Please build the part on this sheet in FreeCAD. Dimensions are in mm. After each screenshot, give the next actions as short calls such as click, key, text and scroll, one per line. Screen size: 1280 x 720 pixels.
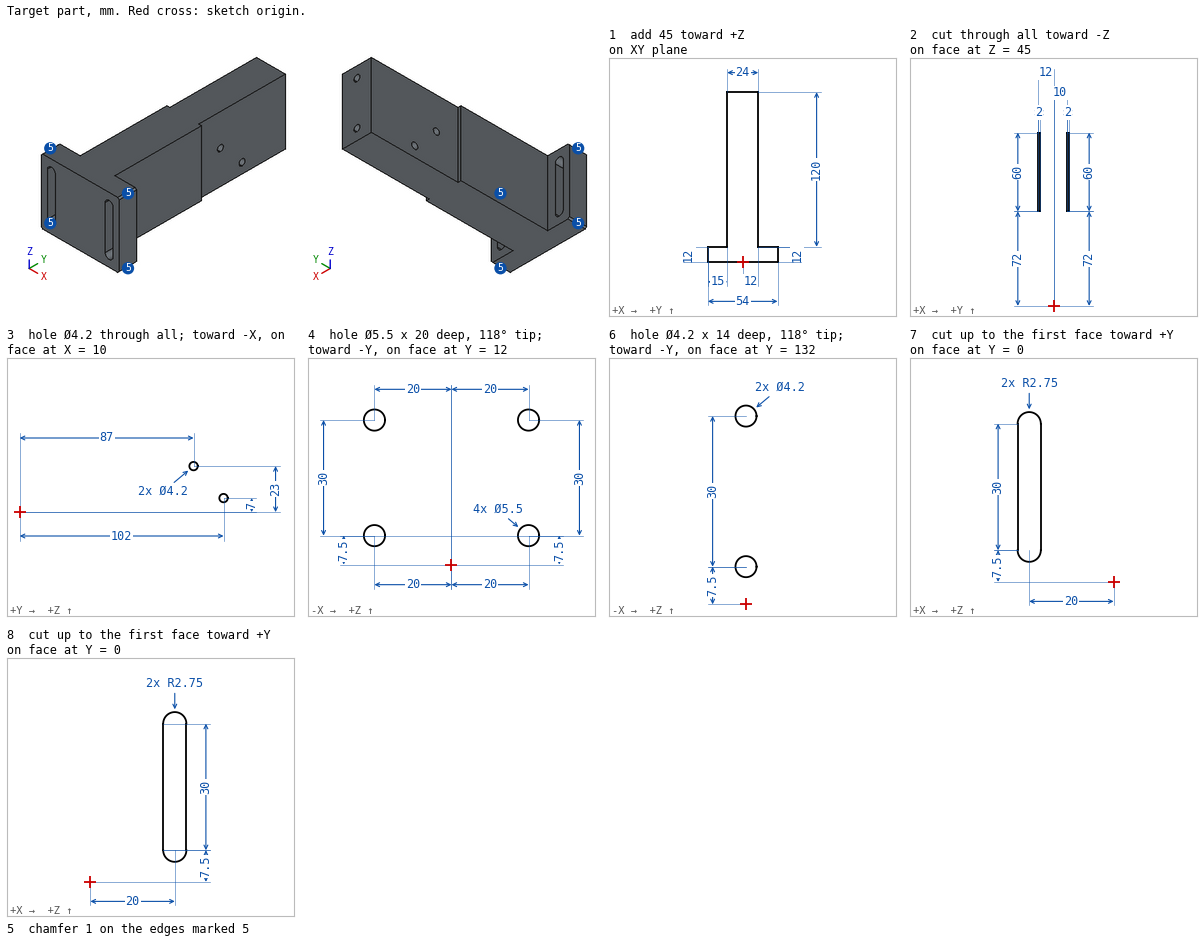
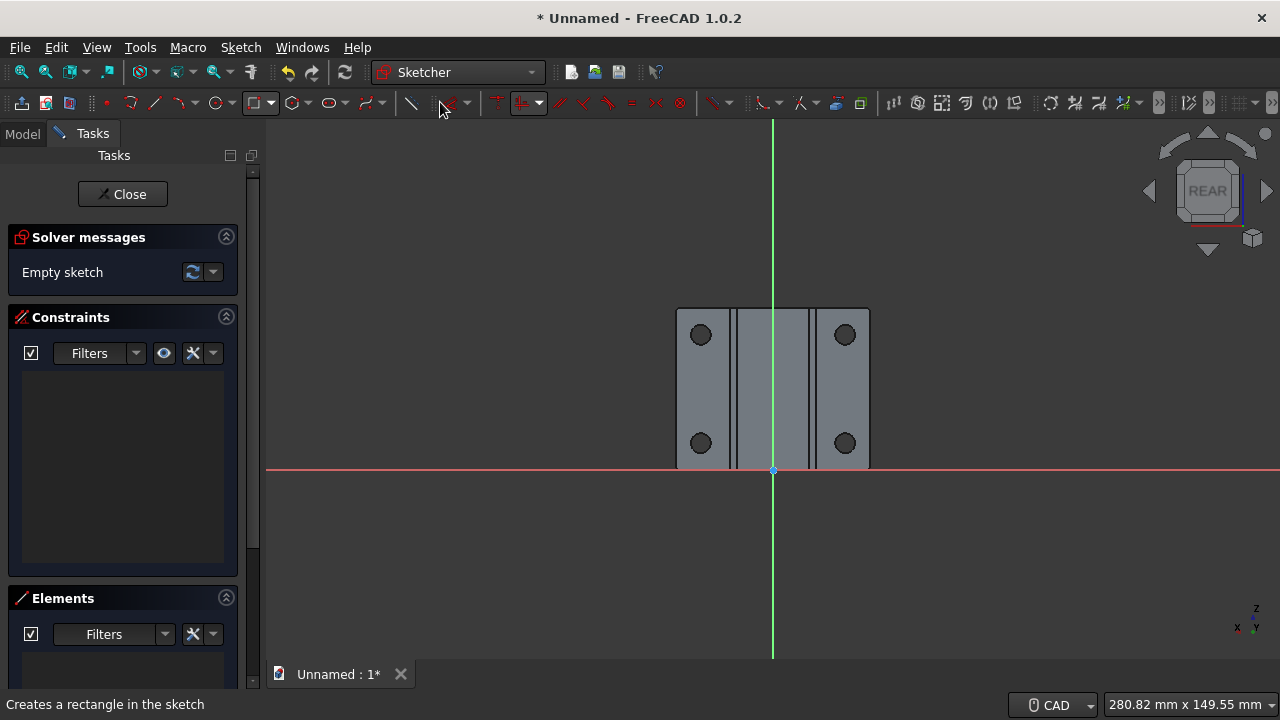
scroll(829, 407, up, 4)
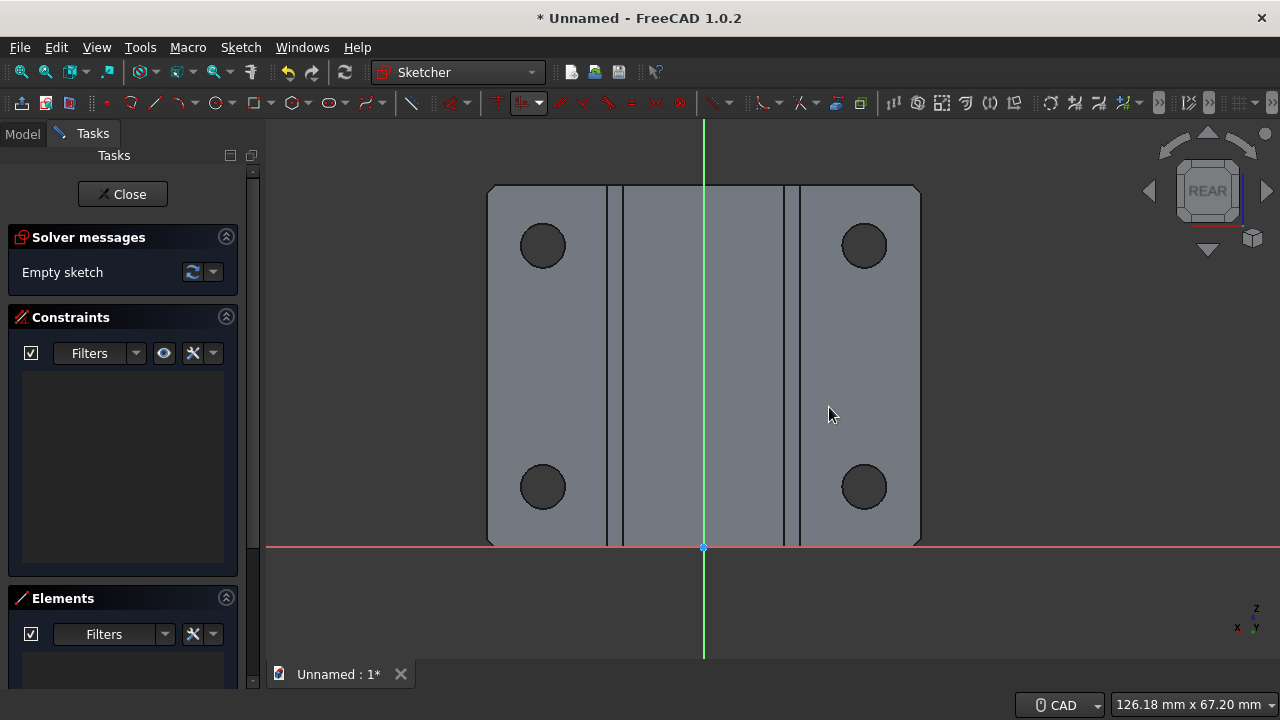
click(216, 104)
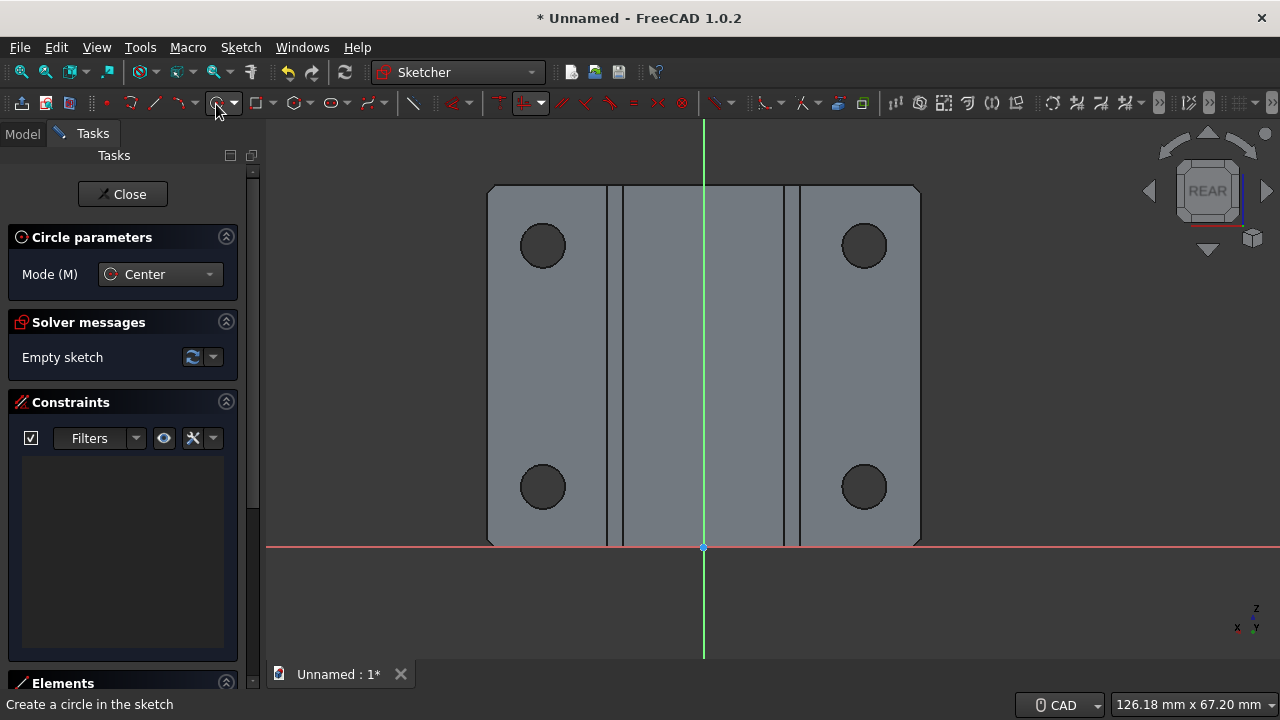
scroll(704, 246, up, 2)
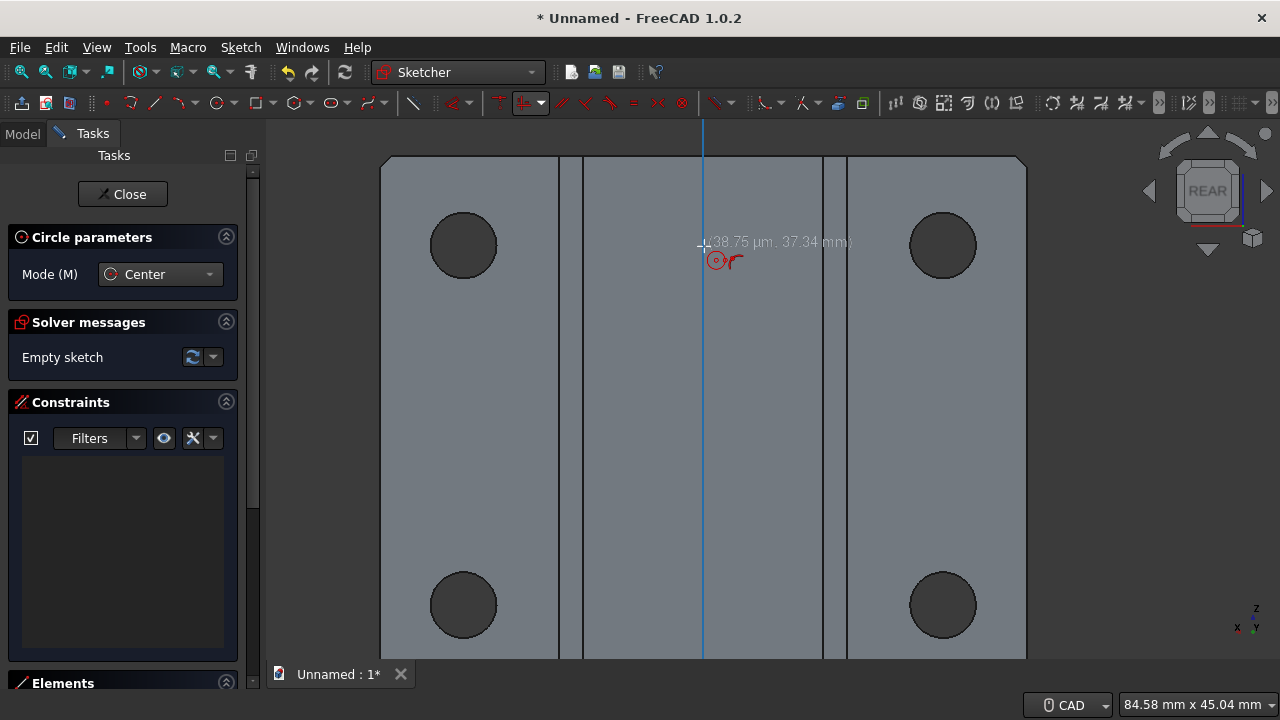
click(703, 246)
move(721, 228)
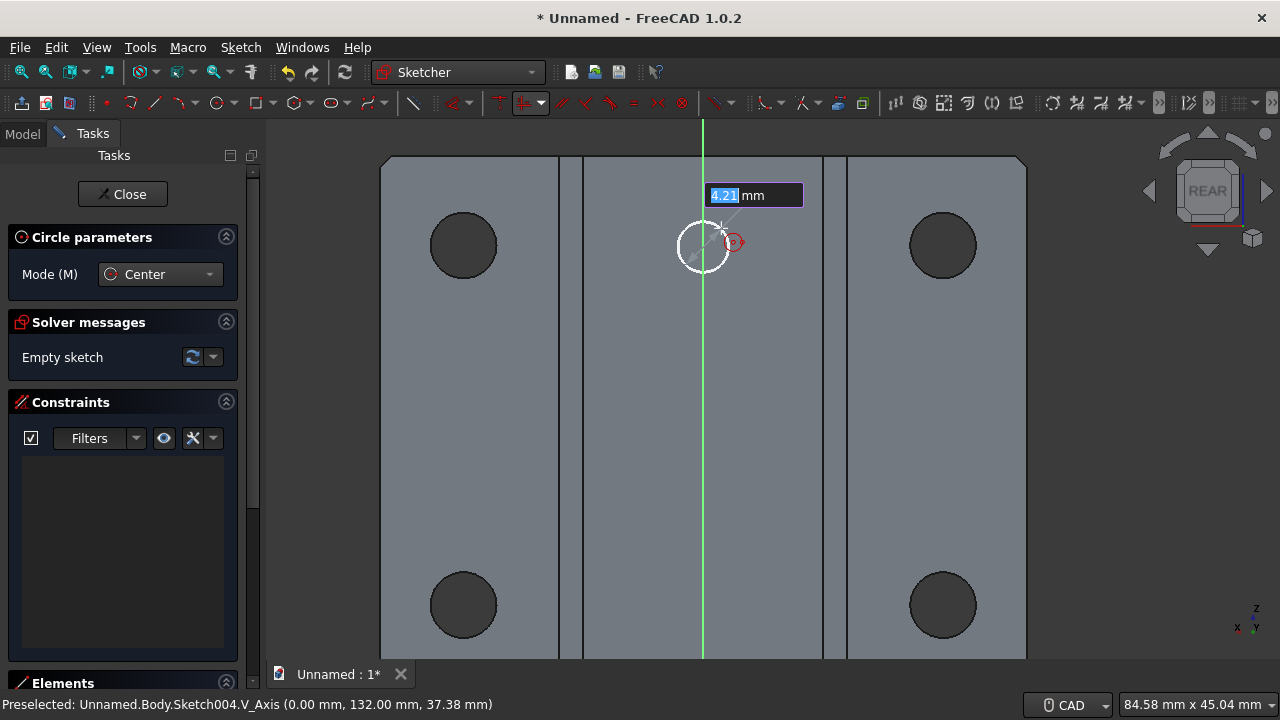
text(4.2)
key(Return)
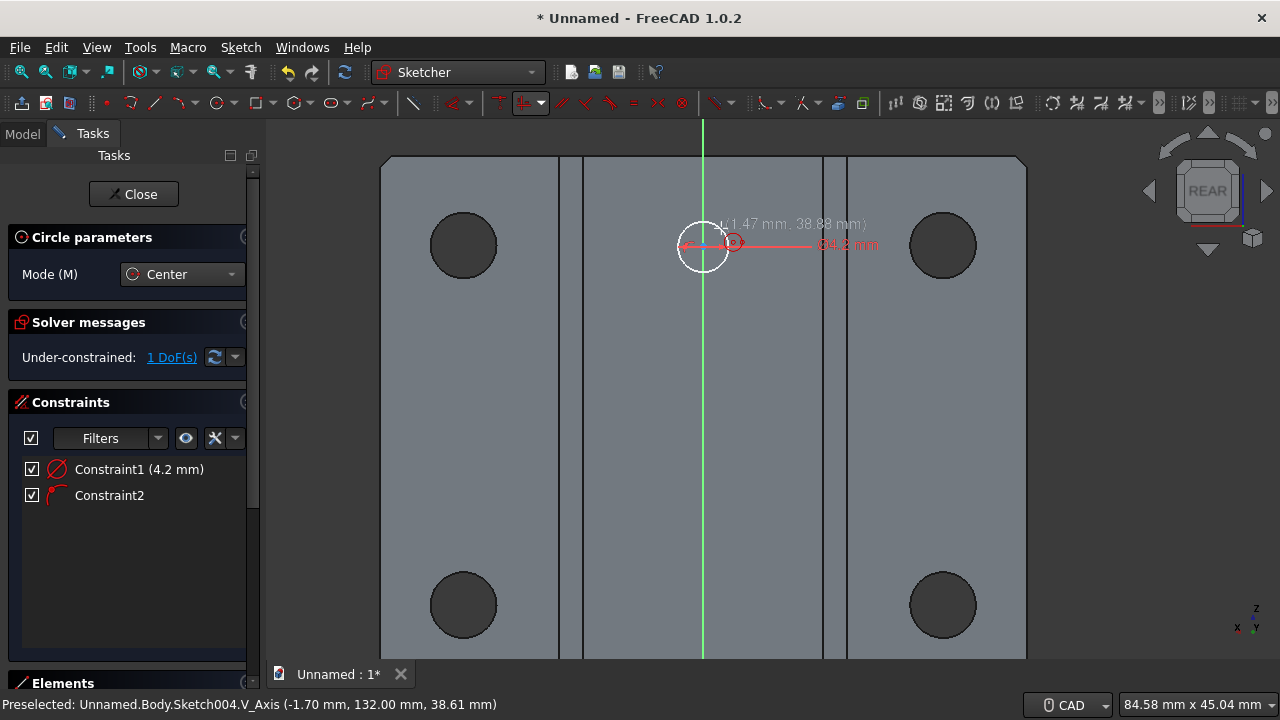
click(703, 605)
move(721, 587)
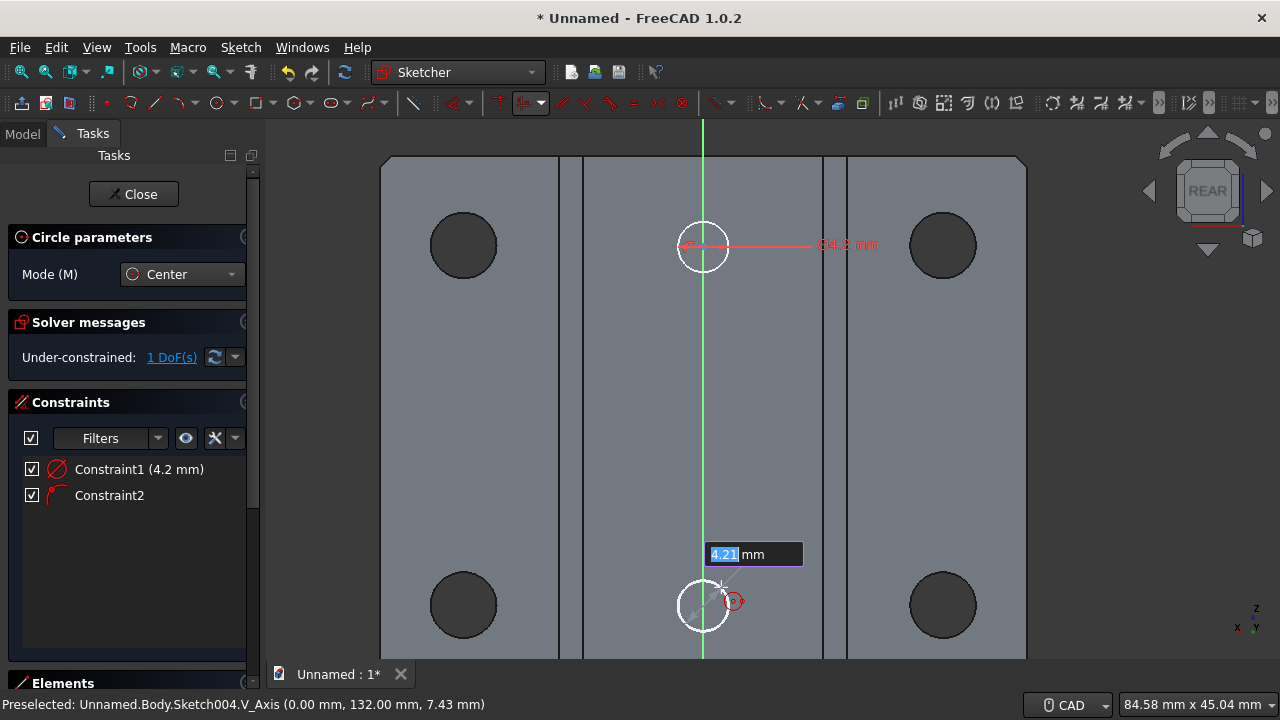
text(4.2)
key(Return)
key(Escape)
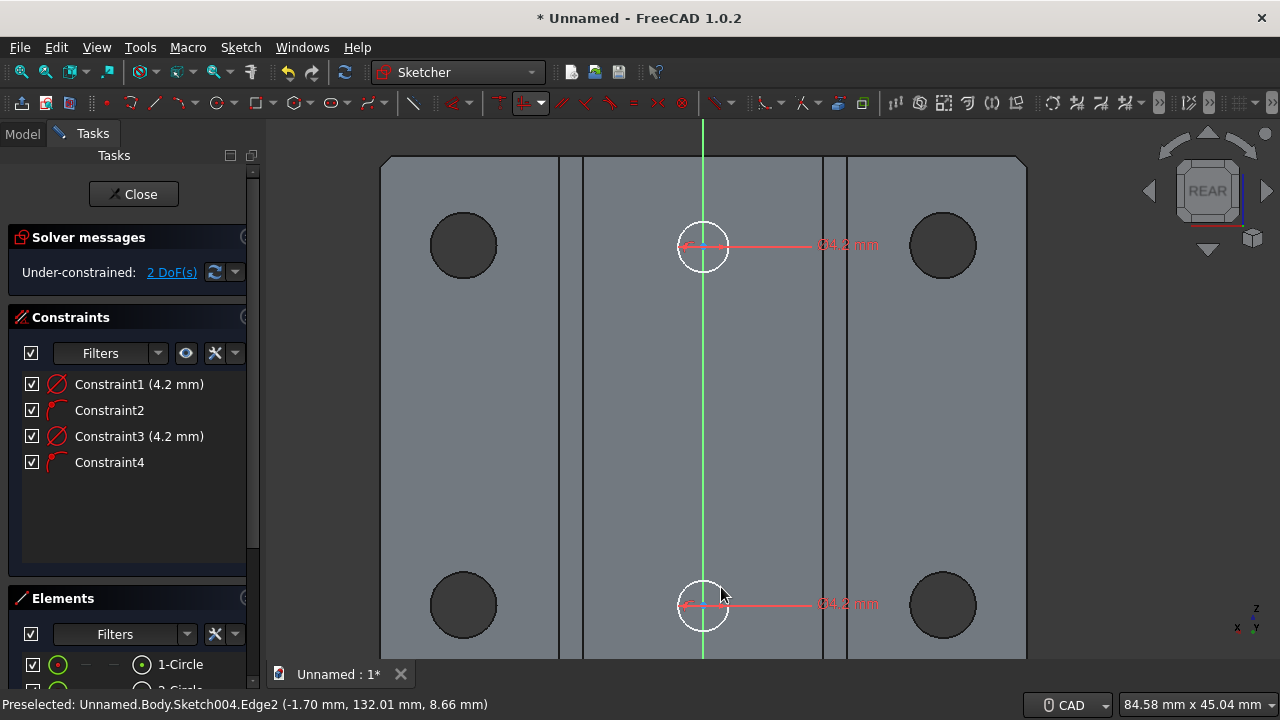
click(452, 104)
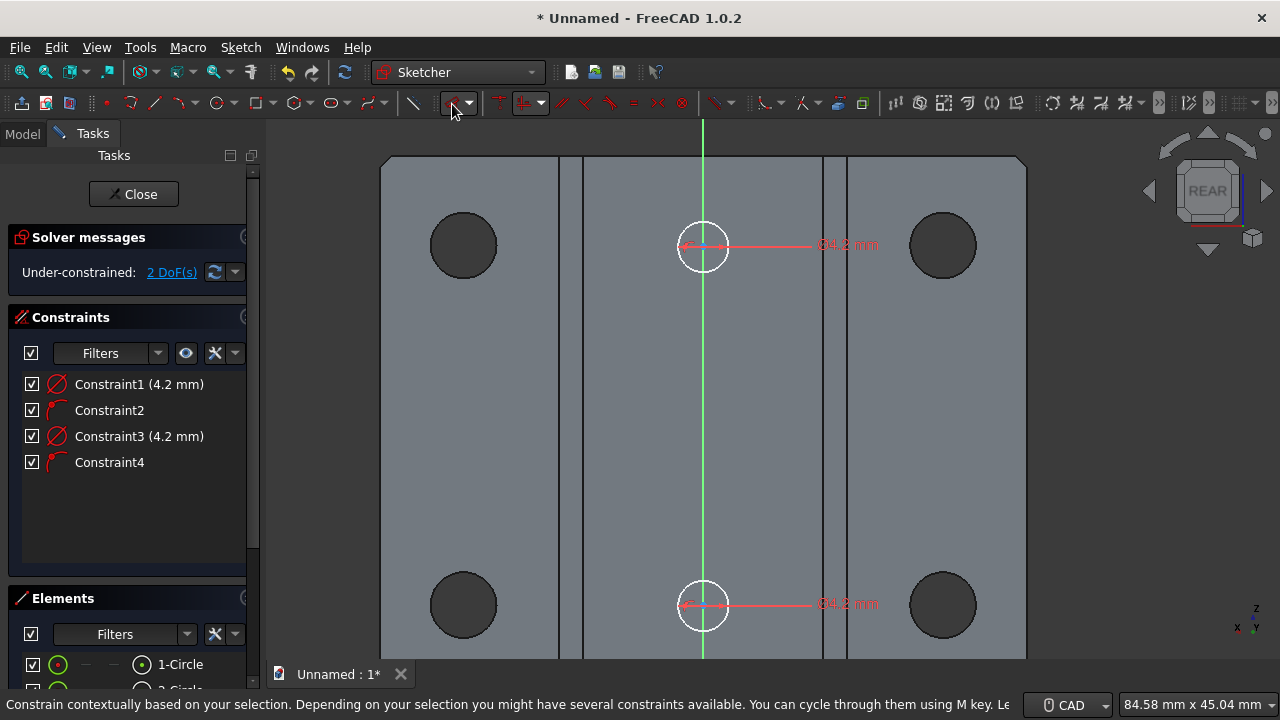
click(703, 606)
click(737, 624)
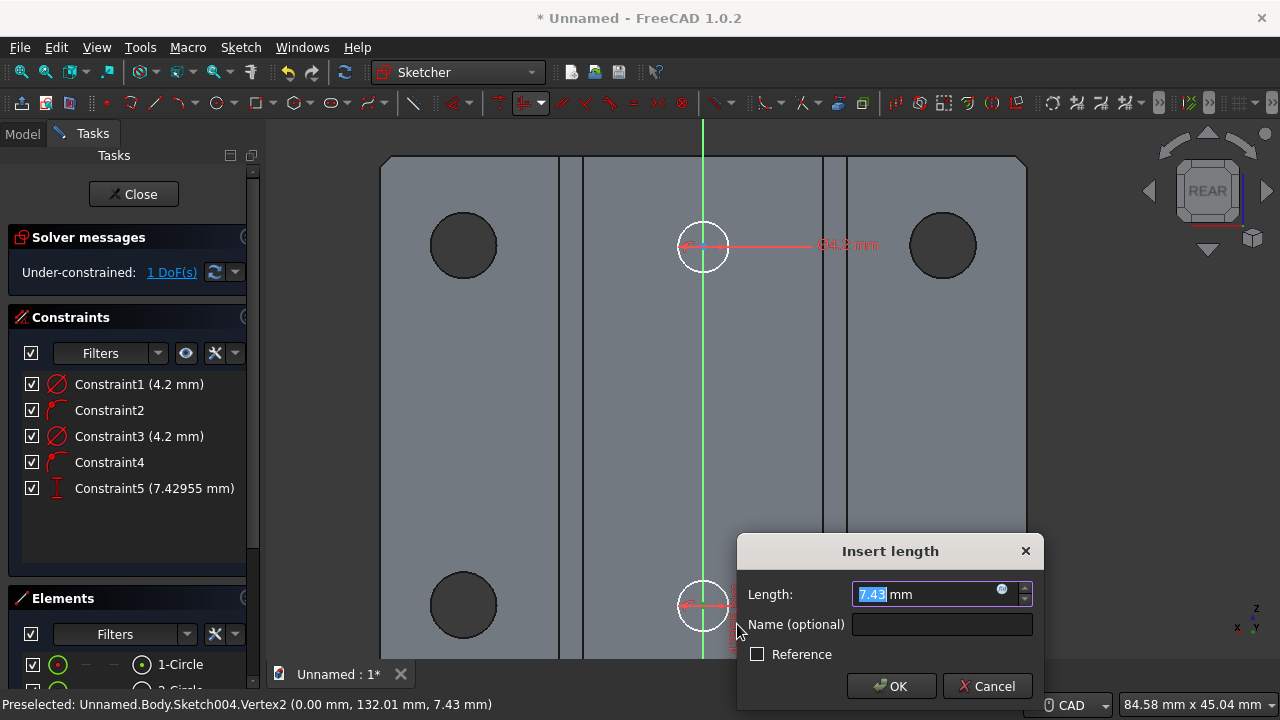
text(7.5)
key(Return)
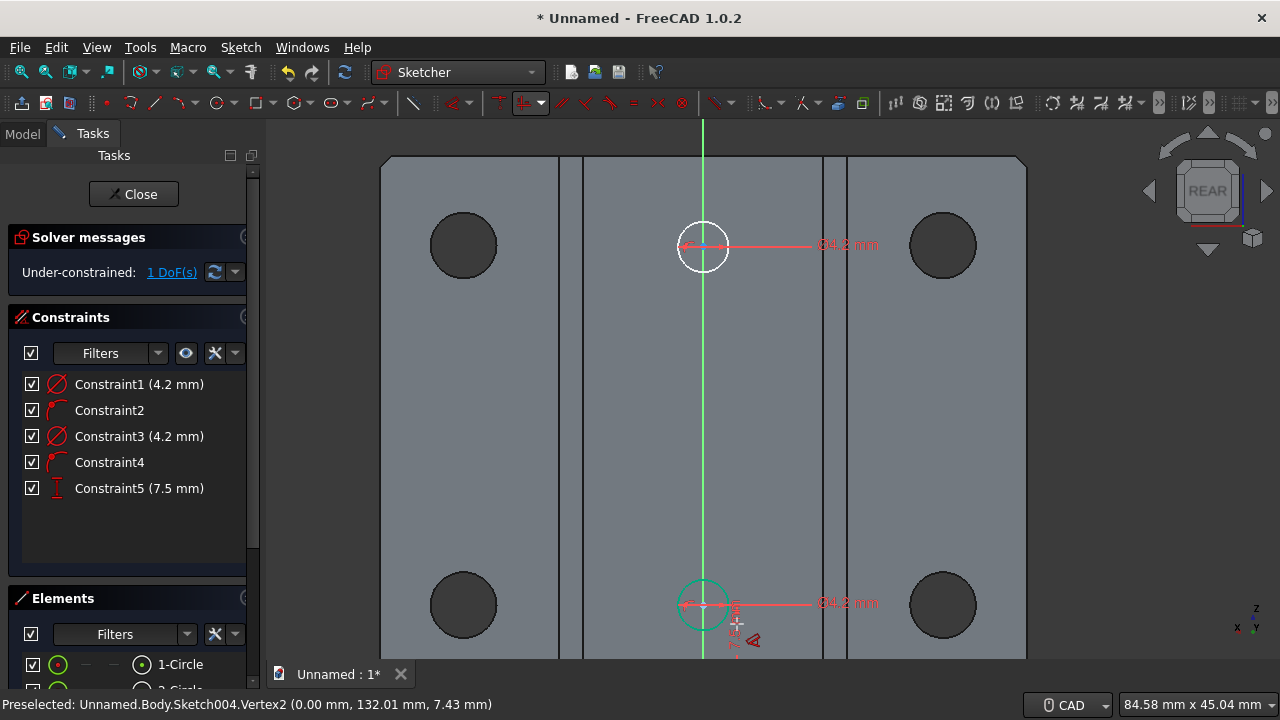
click(703, 247)